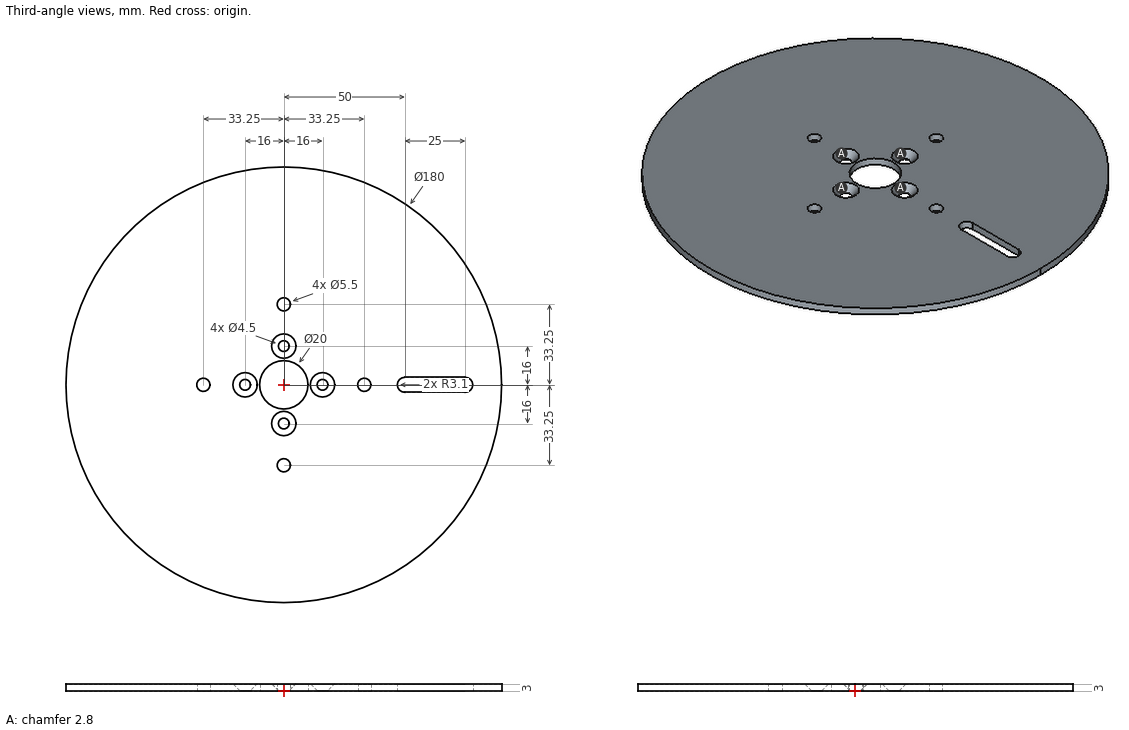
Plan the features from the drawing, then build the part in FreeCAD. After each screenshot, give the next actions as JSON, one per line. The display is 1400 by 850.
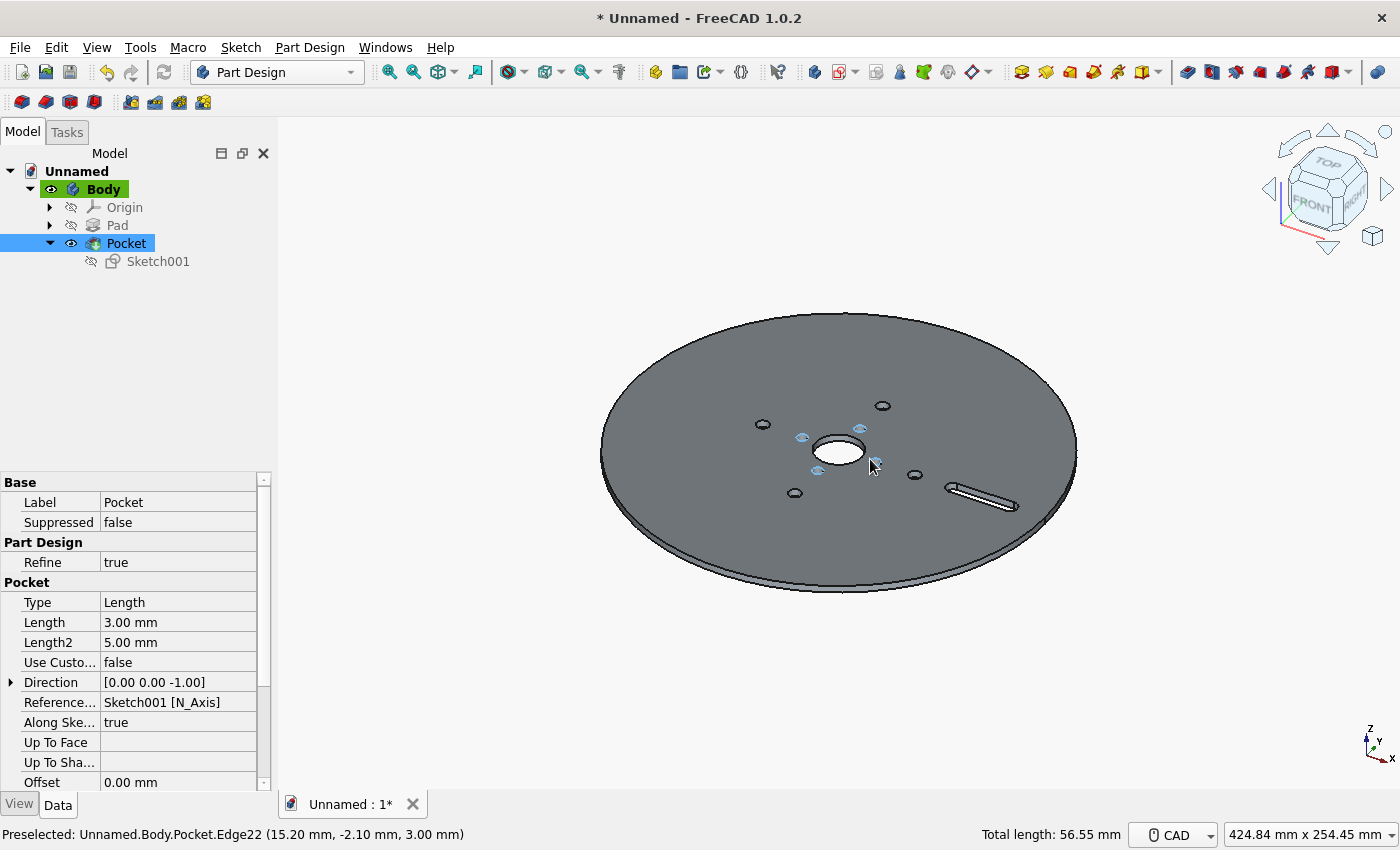
{"action": "left_click", "coordinate": [46, 102]}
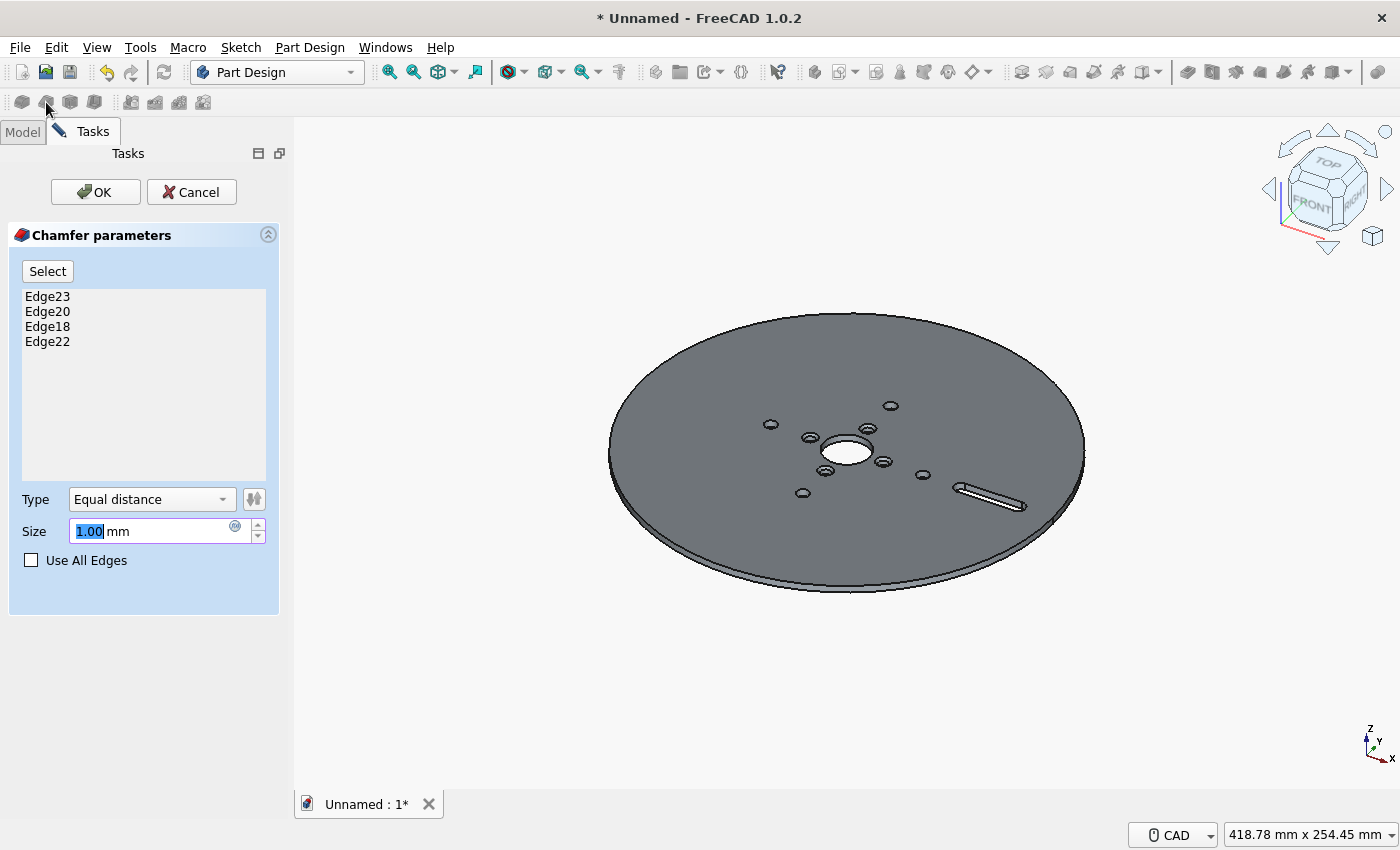
{"action": "type", "text": "2.8"}
{"action": "key", "text": "Tab"}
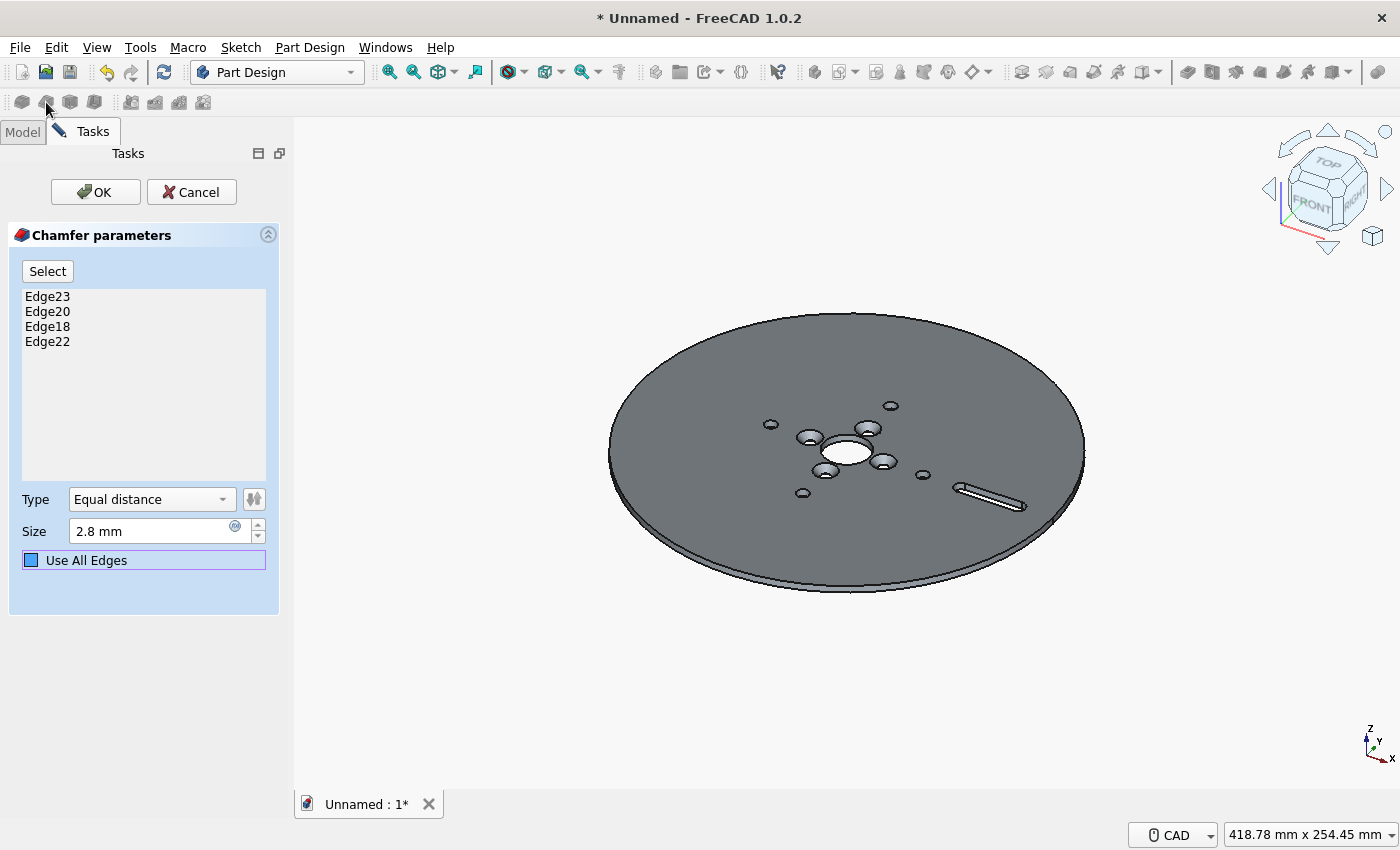
{"action": "left_click", "coordinate": [96, 192]}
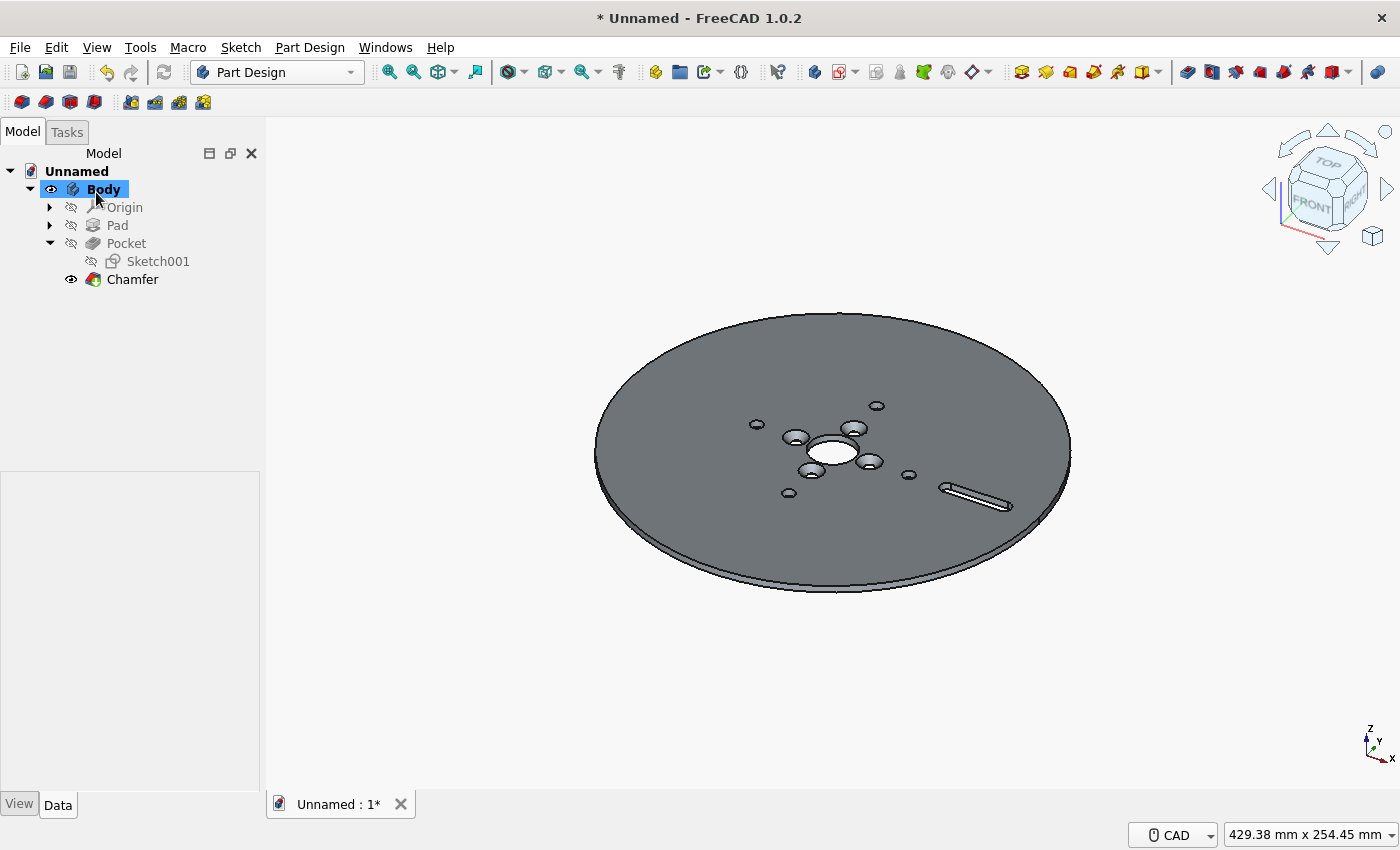
{"action": "key", "text": "0"}